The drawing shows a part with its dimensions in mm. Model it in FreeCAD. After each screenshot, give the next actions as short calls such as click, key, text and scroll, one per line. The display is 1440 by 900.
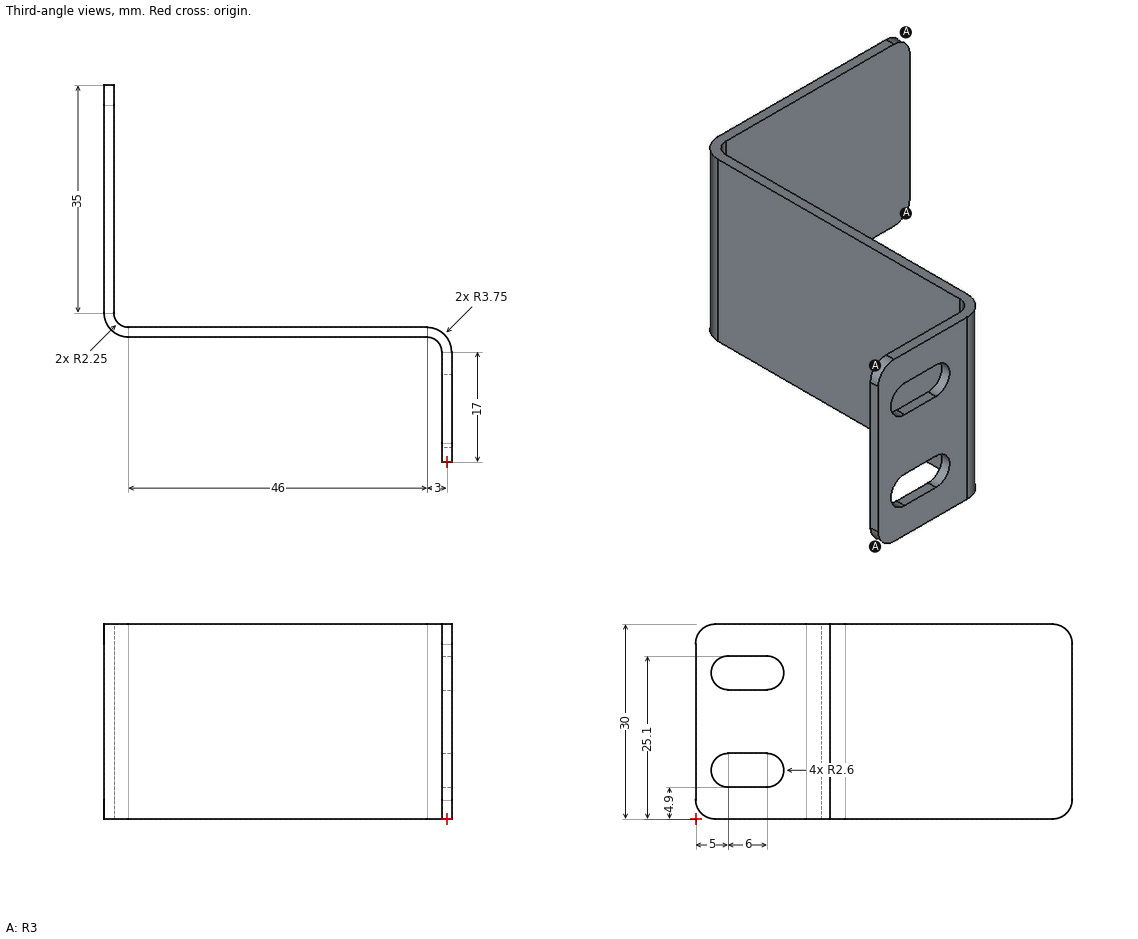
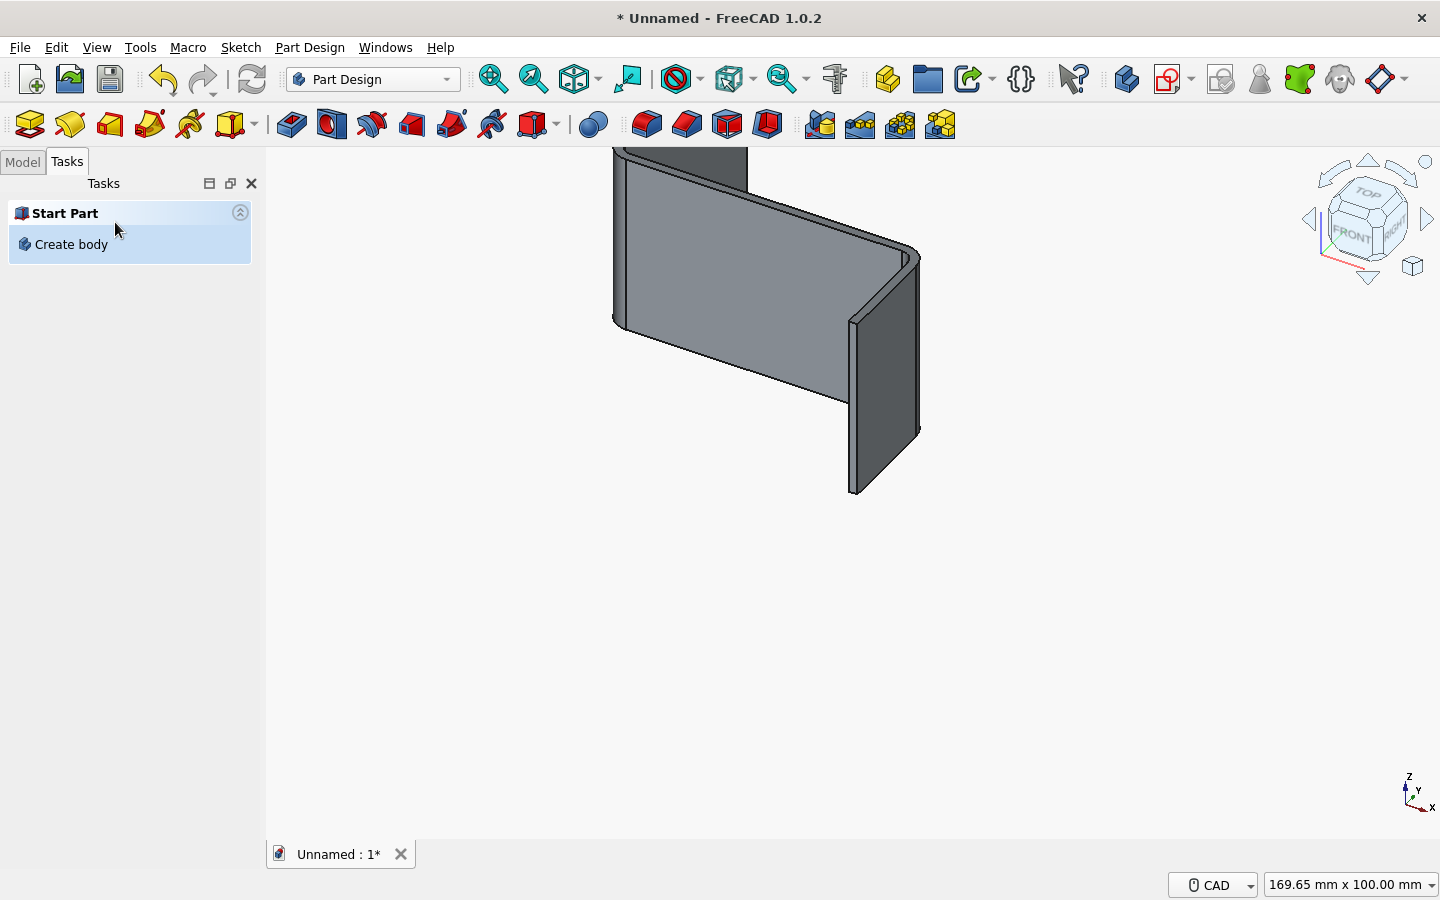
key(v)
key(f)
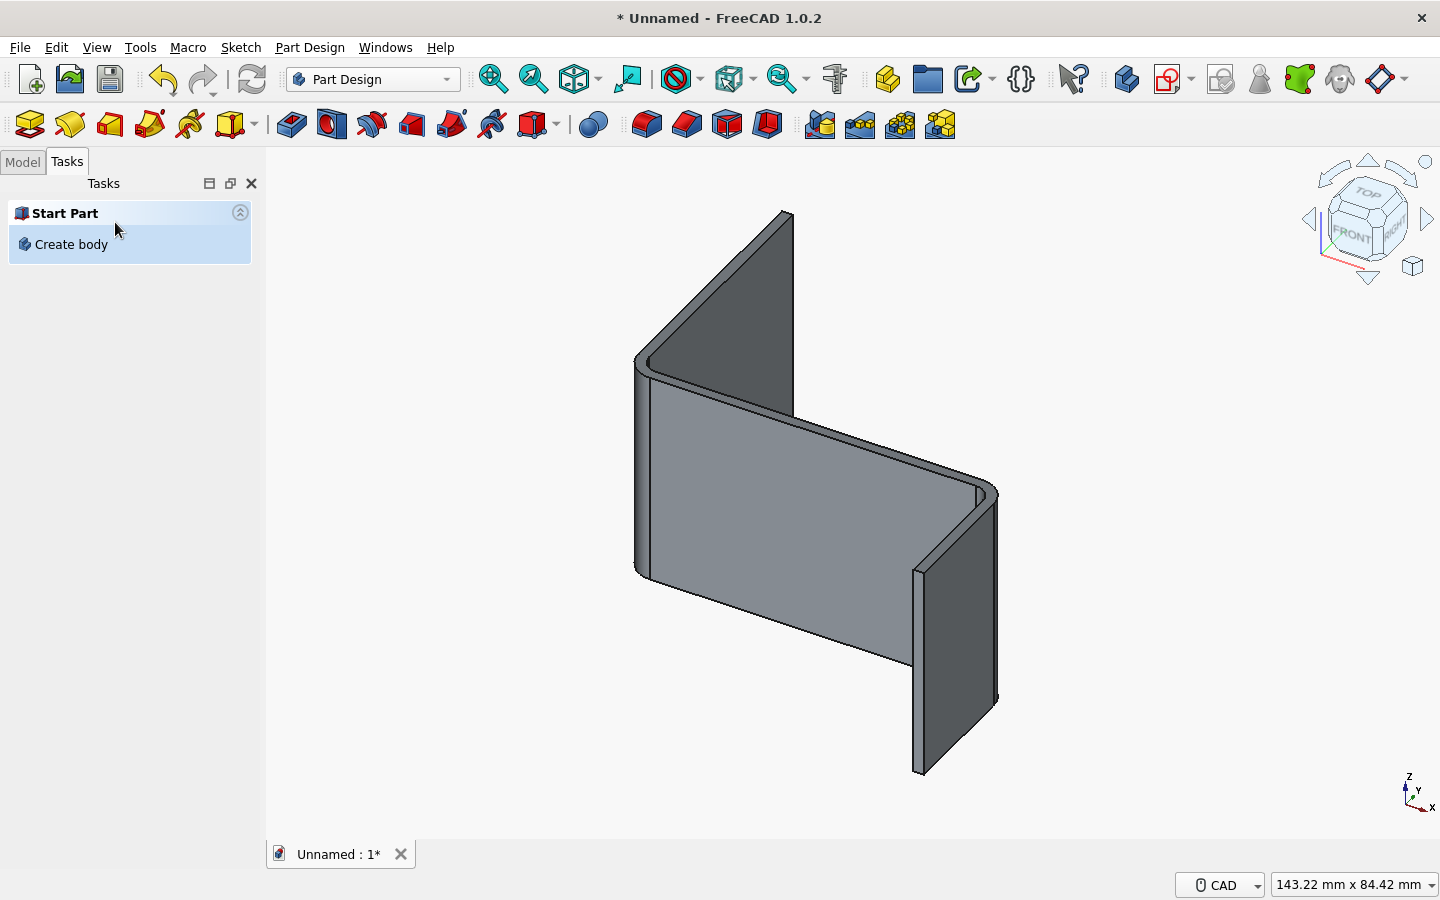
click(918, 570)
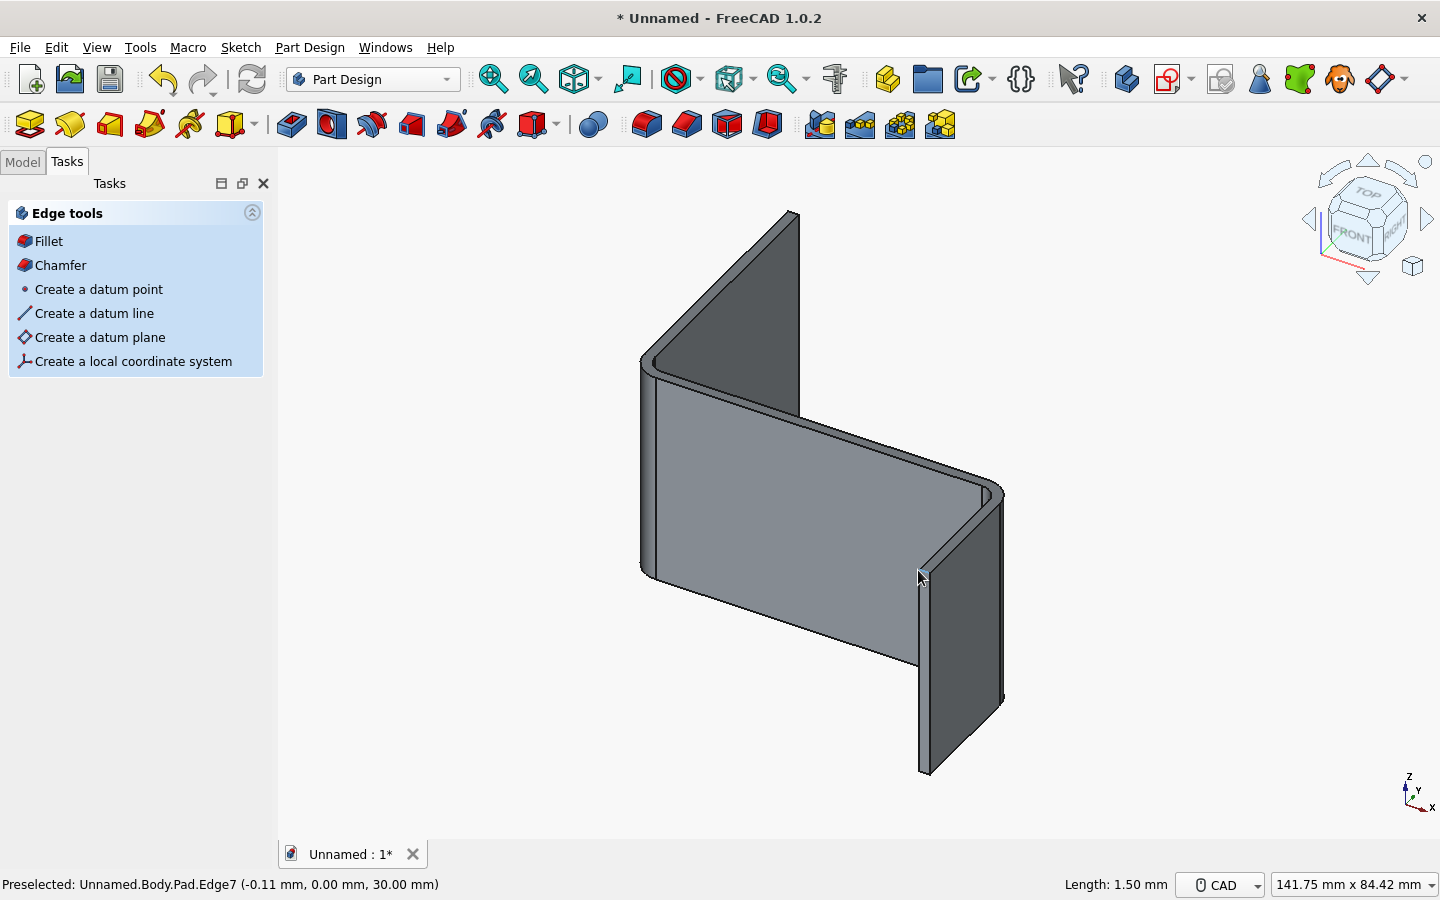
scroll(925, 772, up, 6)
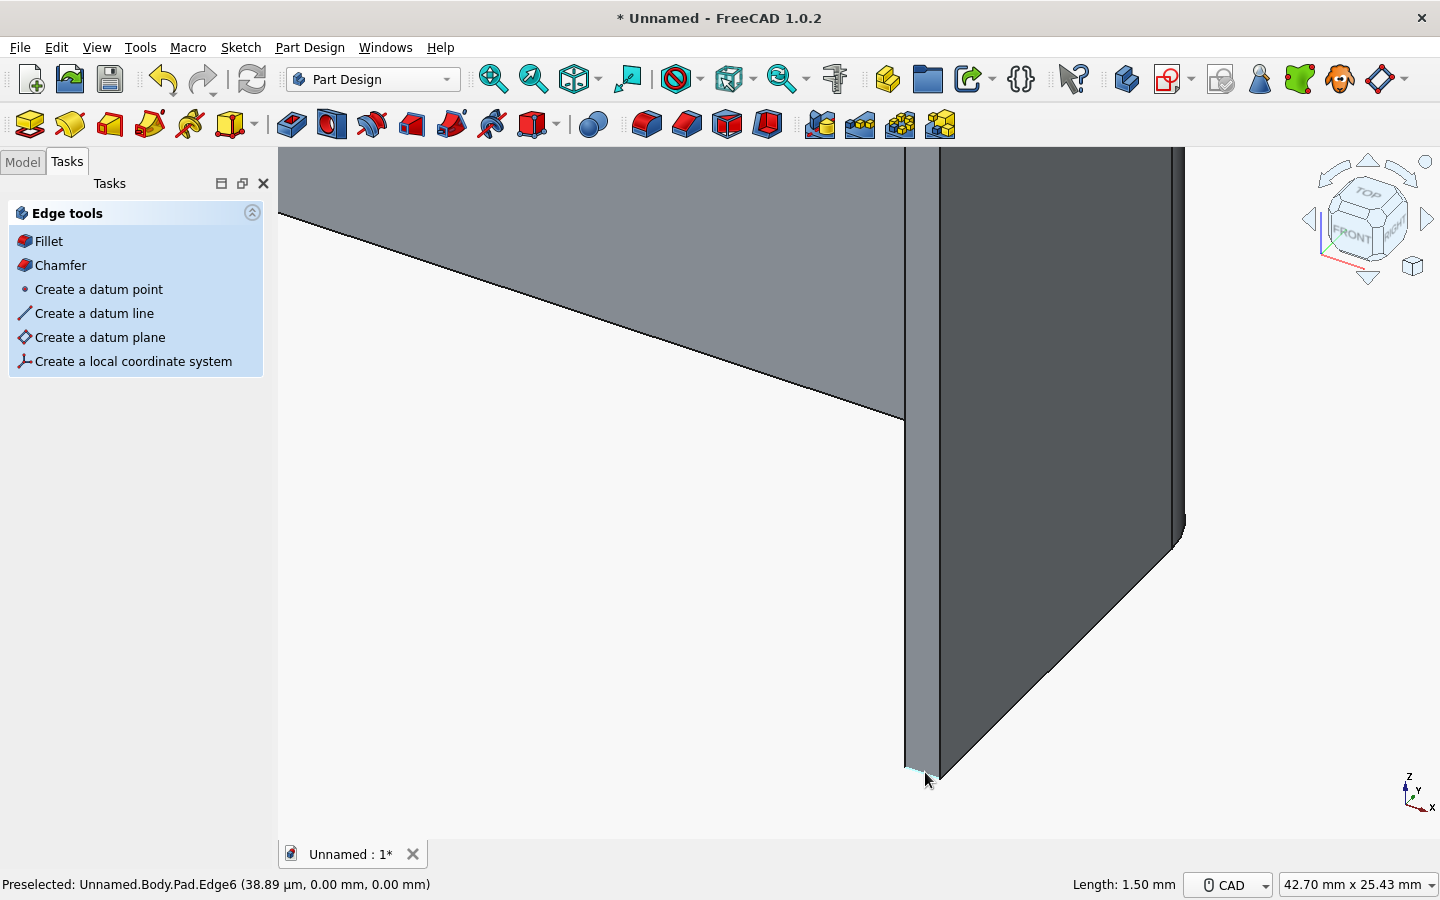
key(v)
key(f)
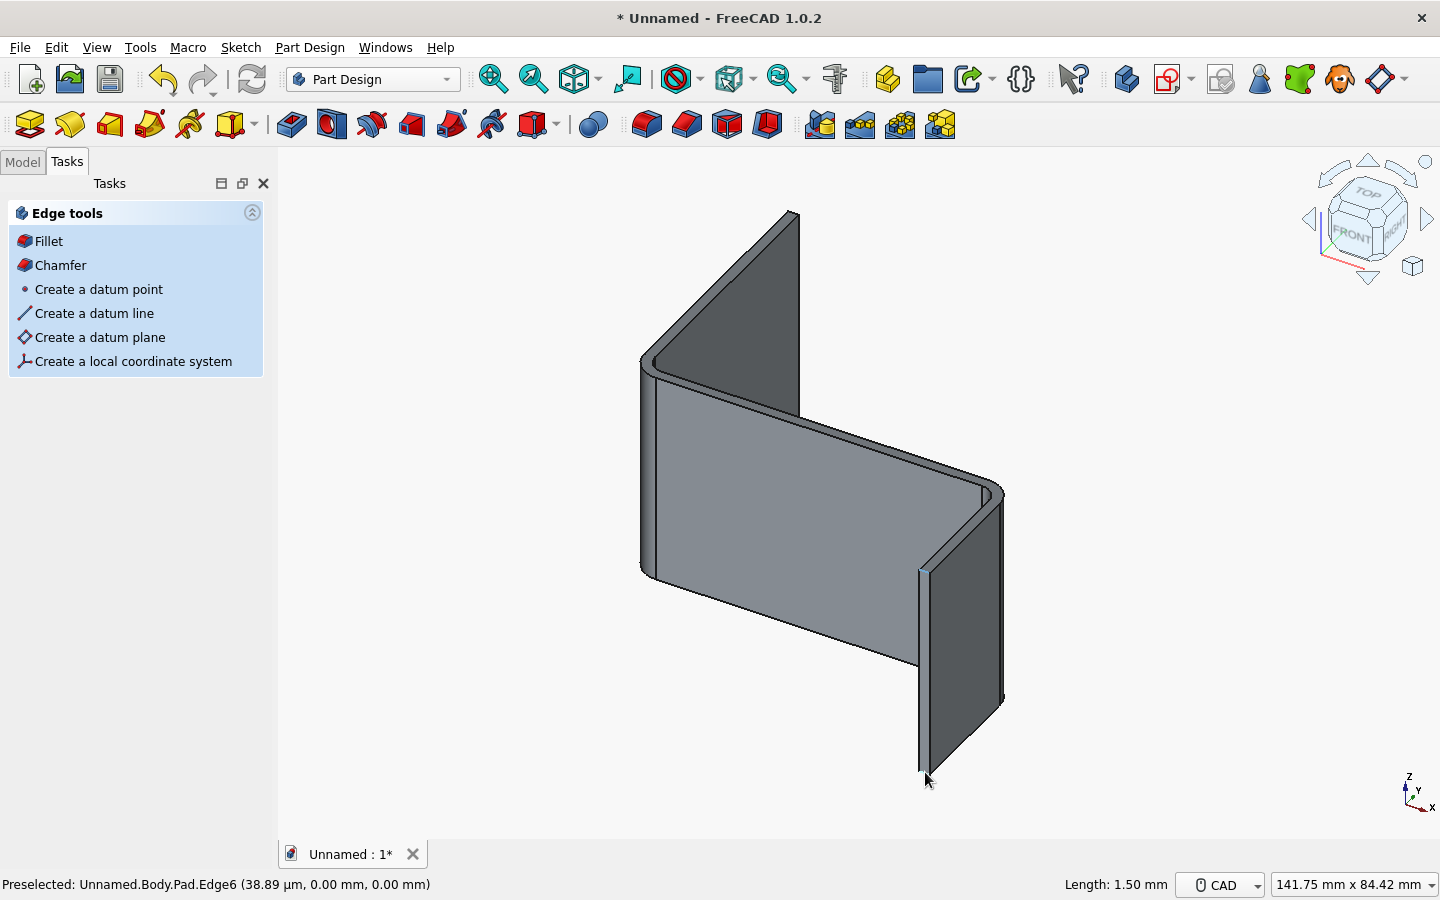
key(0)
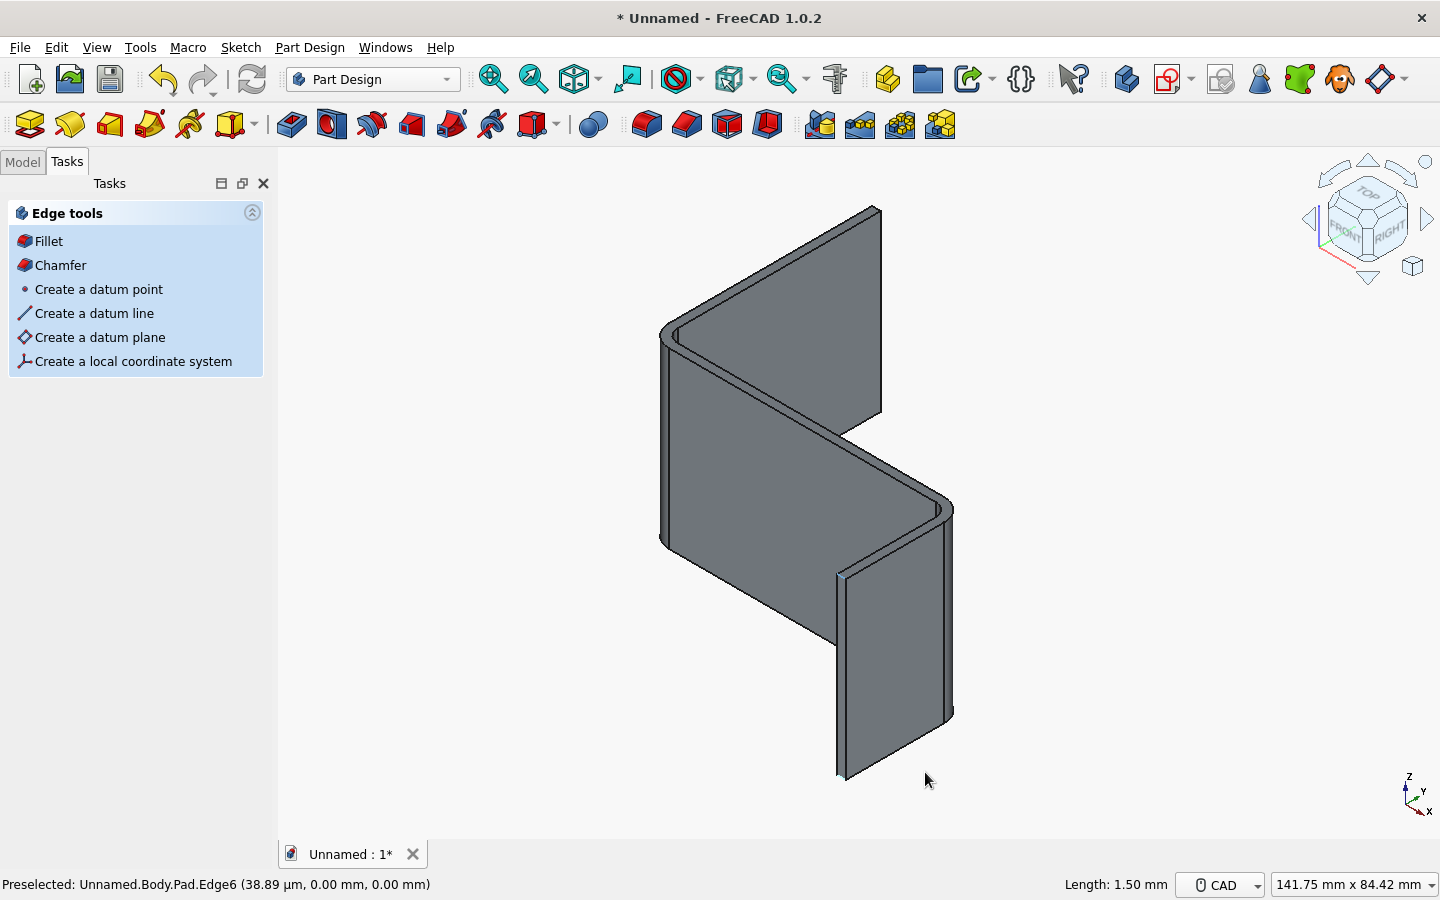
scroll(842, 776, up, 6)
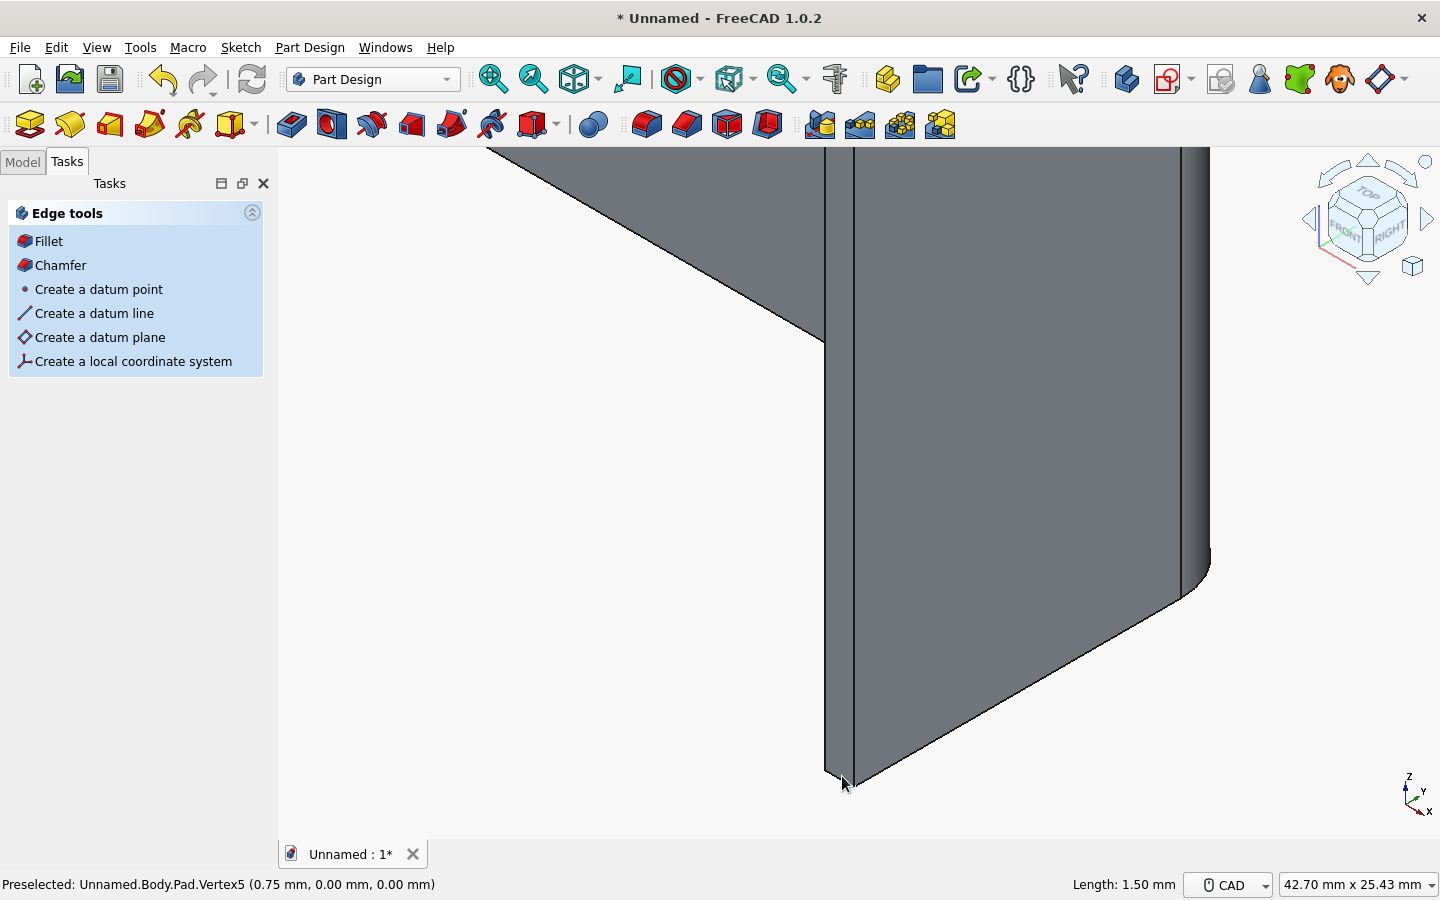
key(v)
key(f)